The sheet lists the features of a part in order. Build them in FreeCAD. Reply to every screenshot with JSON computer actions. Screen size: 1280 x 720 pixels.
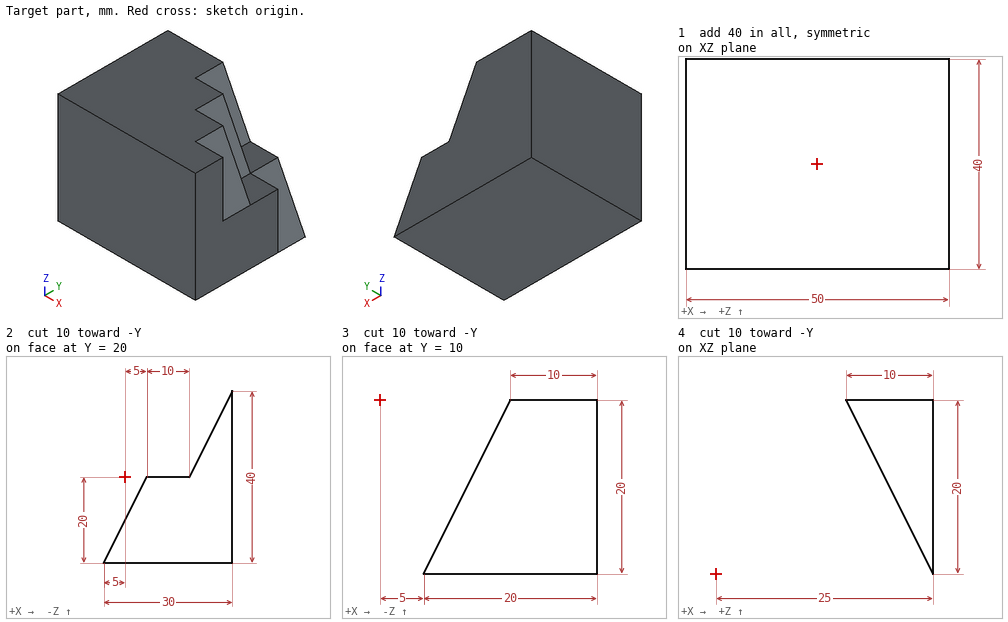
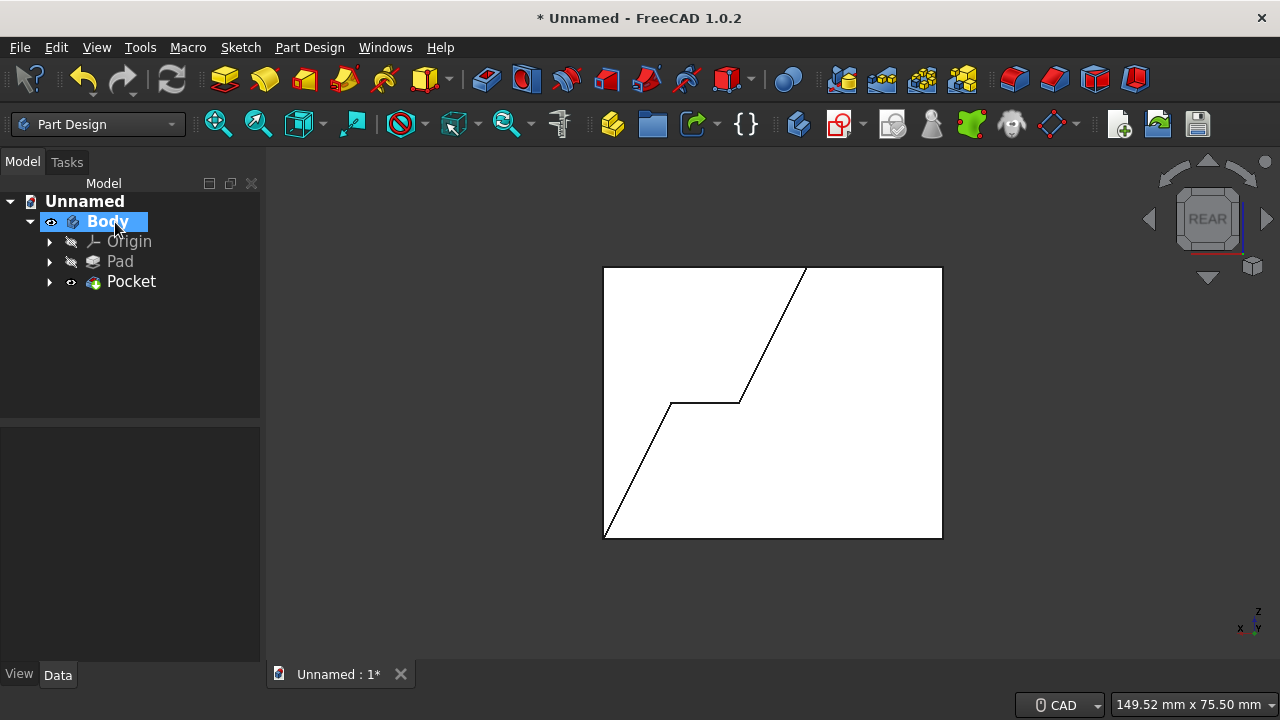
{"action": "left_click", "coordinate": [676, 324]}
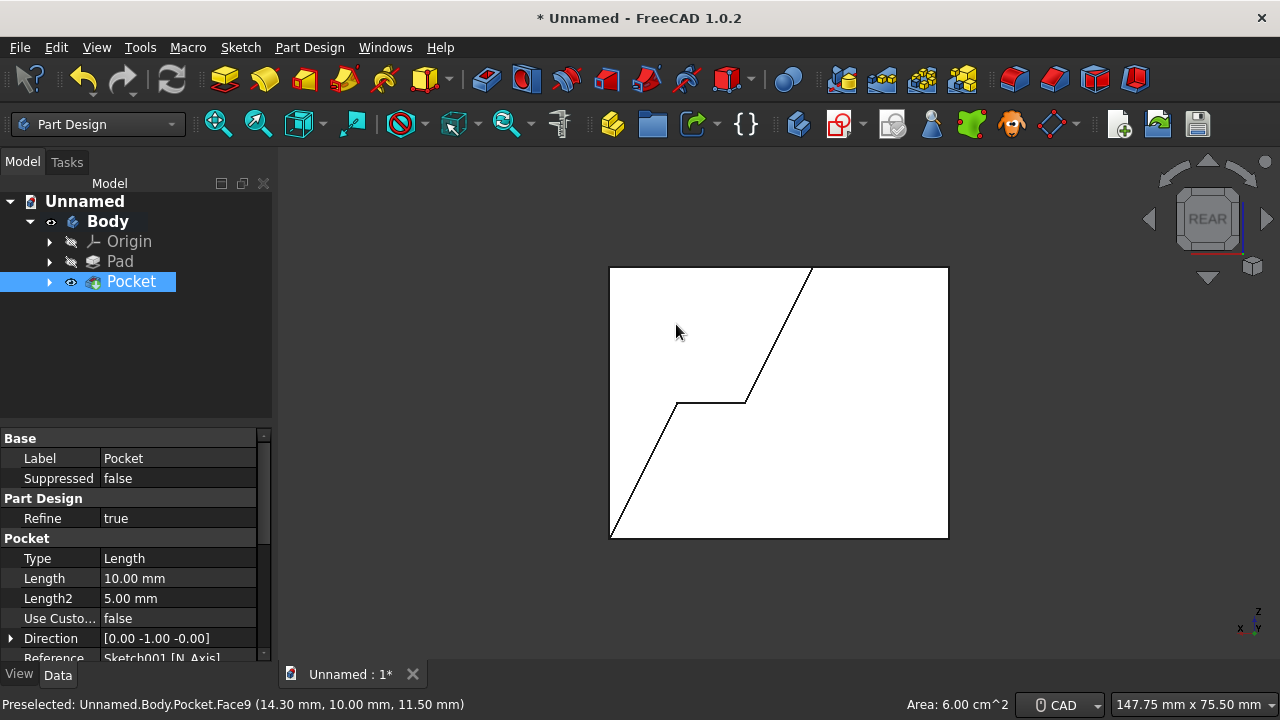
{"action": "left_click", "coordinate": [840, 124]}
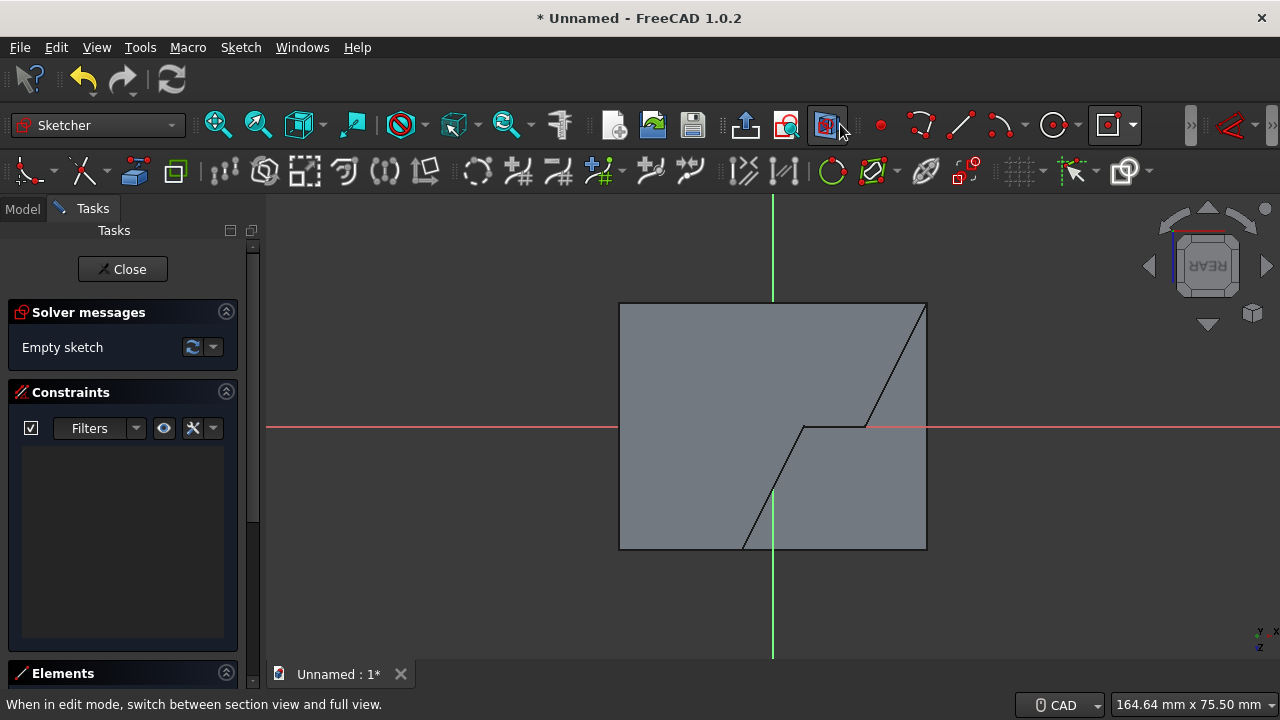
{"action": "scroll", "coordinate": [969, 538], "scroll_direction": "up", "scroll_amount": 4}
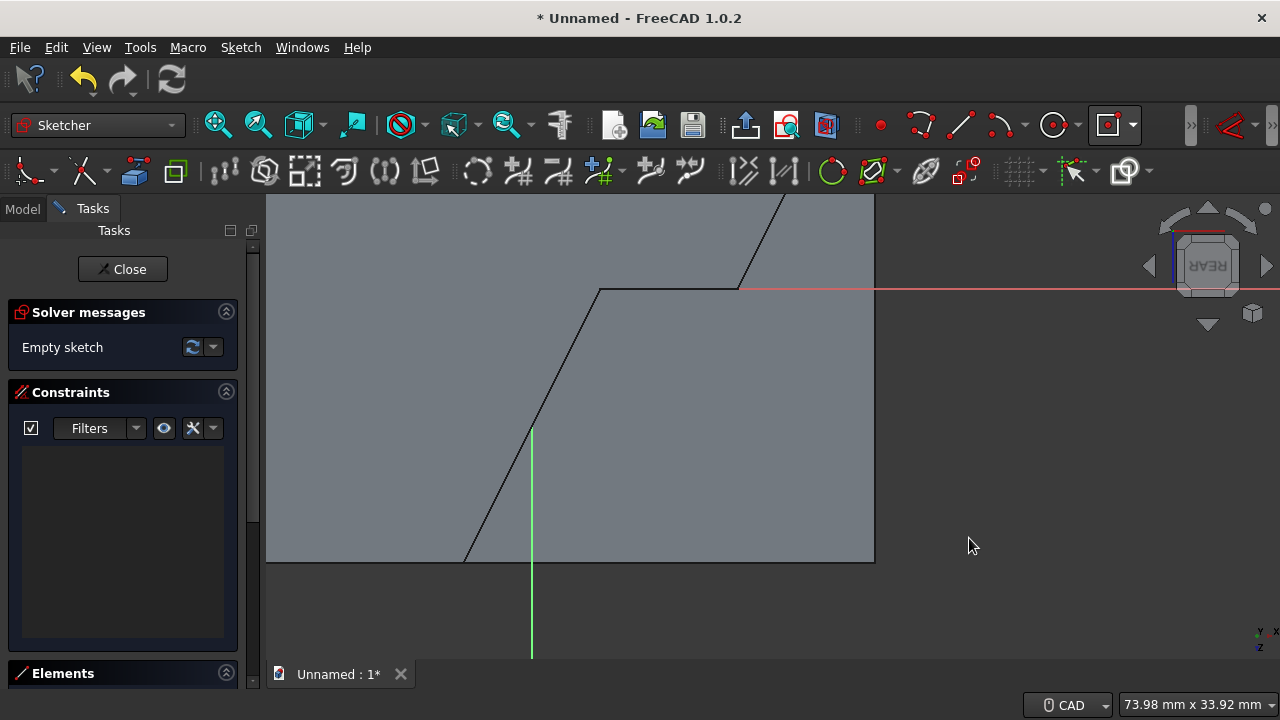
{"action": "left_click", "coordinate": [922, 126]}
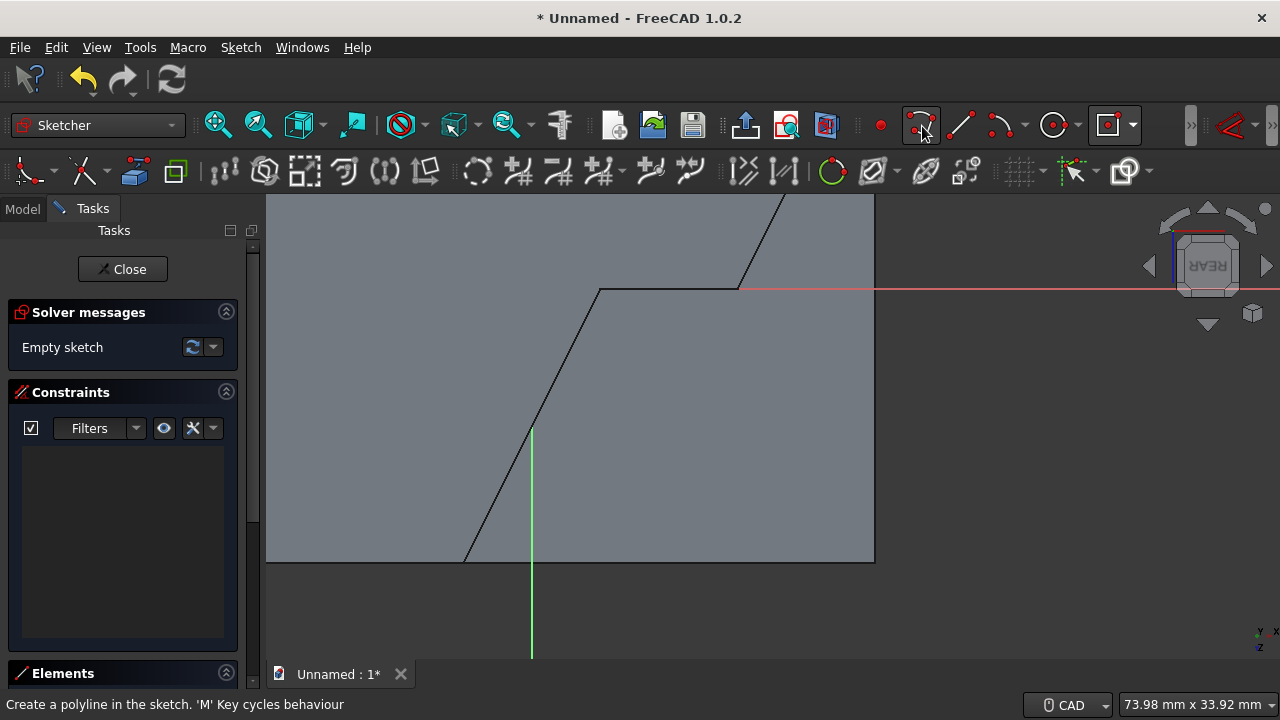
{"action": "left_click", "coordinate": [738, 289]}
{"action": "left_click", "coordinate": [600, 563]}
{"action": "left_click", "coordinate": [875, 563]}
{"action": "left_click", "coordinate": [875, 298]}
{"action": "left_click", "coordinate": [738, 289]}
{"action": "key", "text": "Escape"}
{"action": "key", "text": "Escape"}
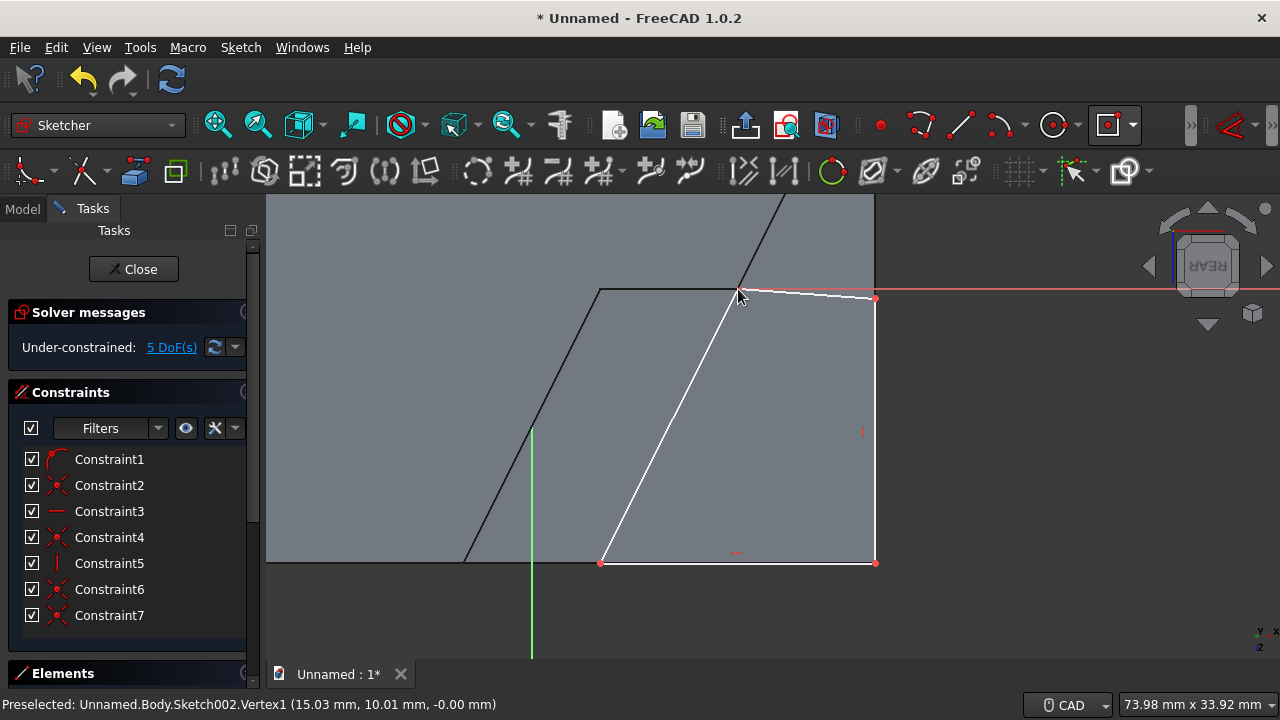
{"action": "left_click", "coordinate": [779, 292]}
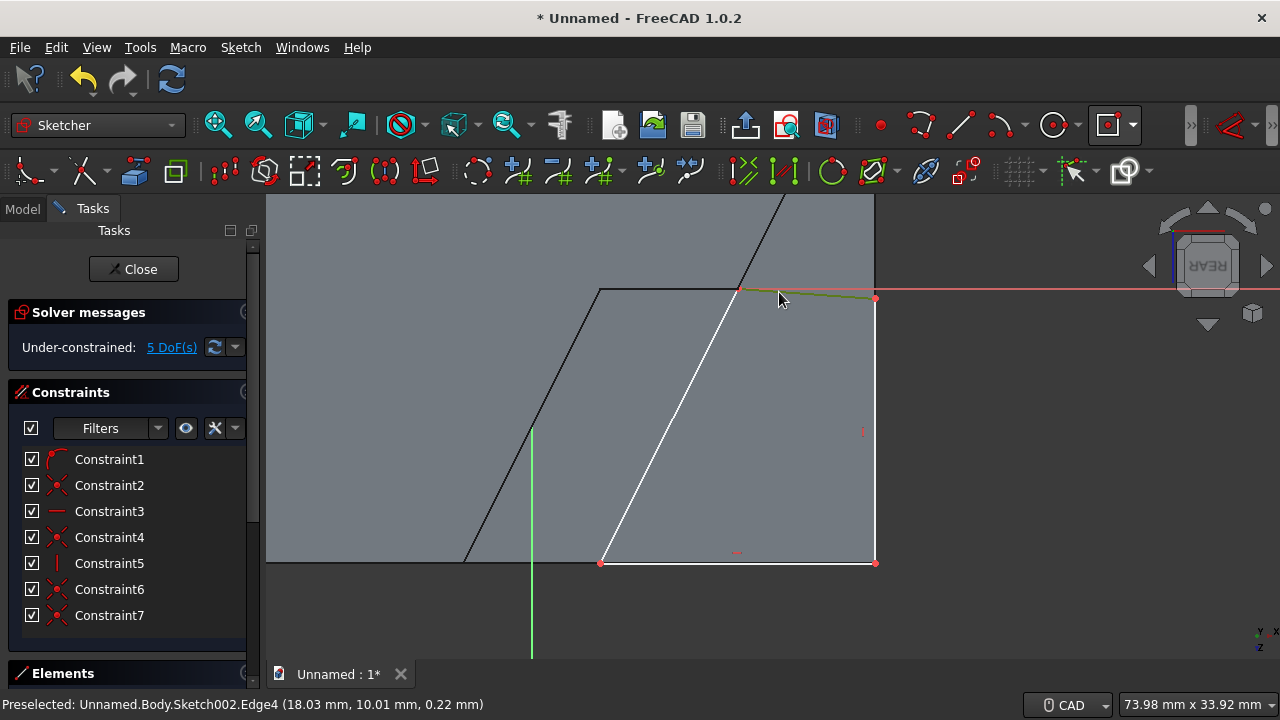
{"action": "key", "text": "h"}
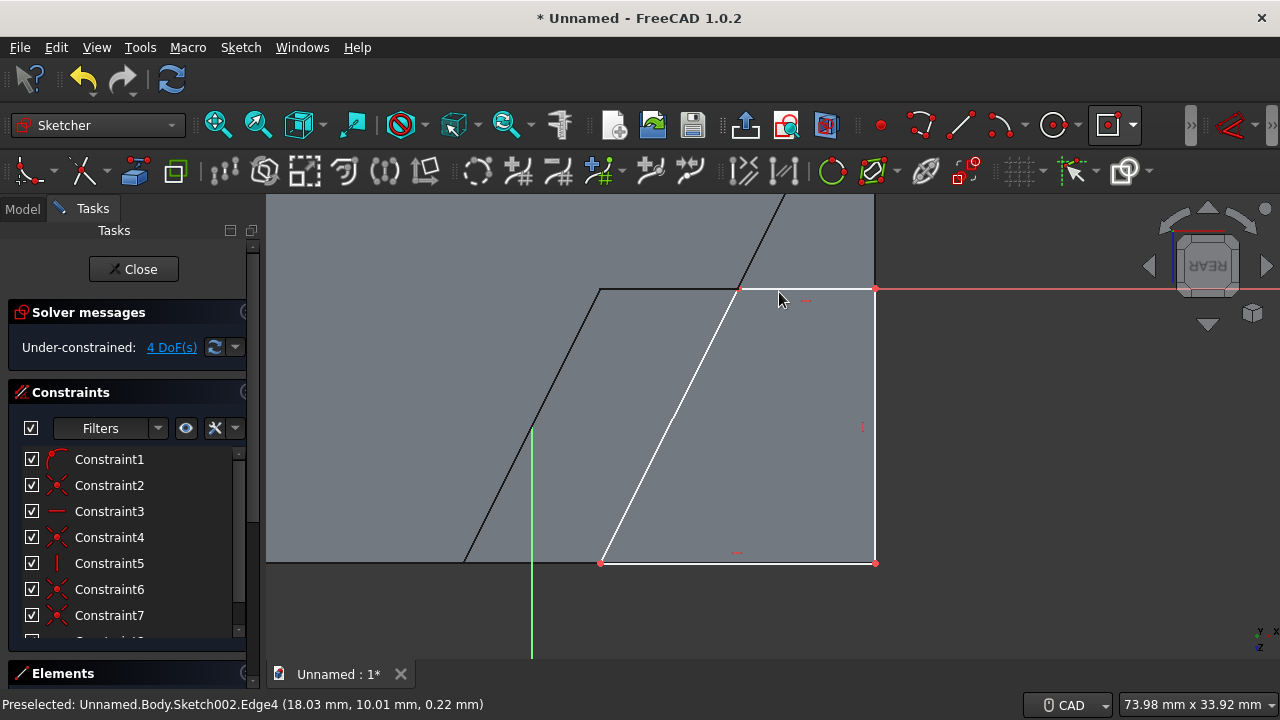
{"action": "left_click", "coordinate": [1230, 126]}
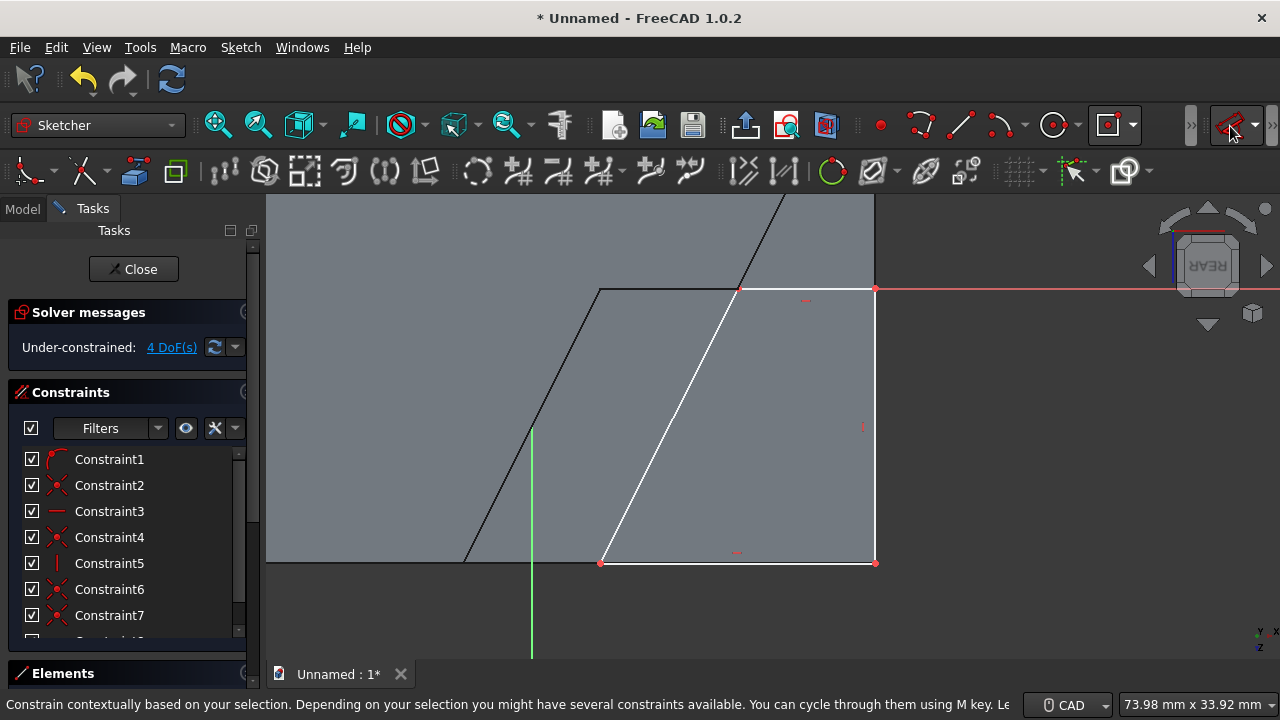
{"action": "left_click", "coordinate": [682, 564]}
{"action": "left_click", "coordinate": [738, 598]}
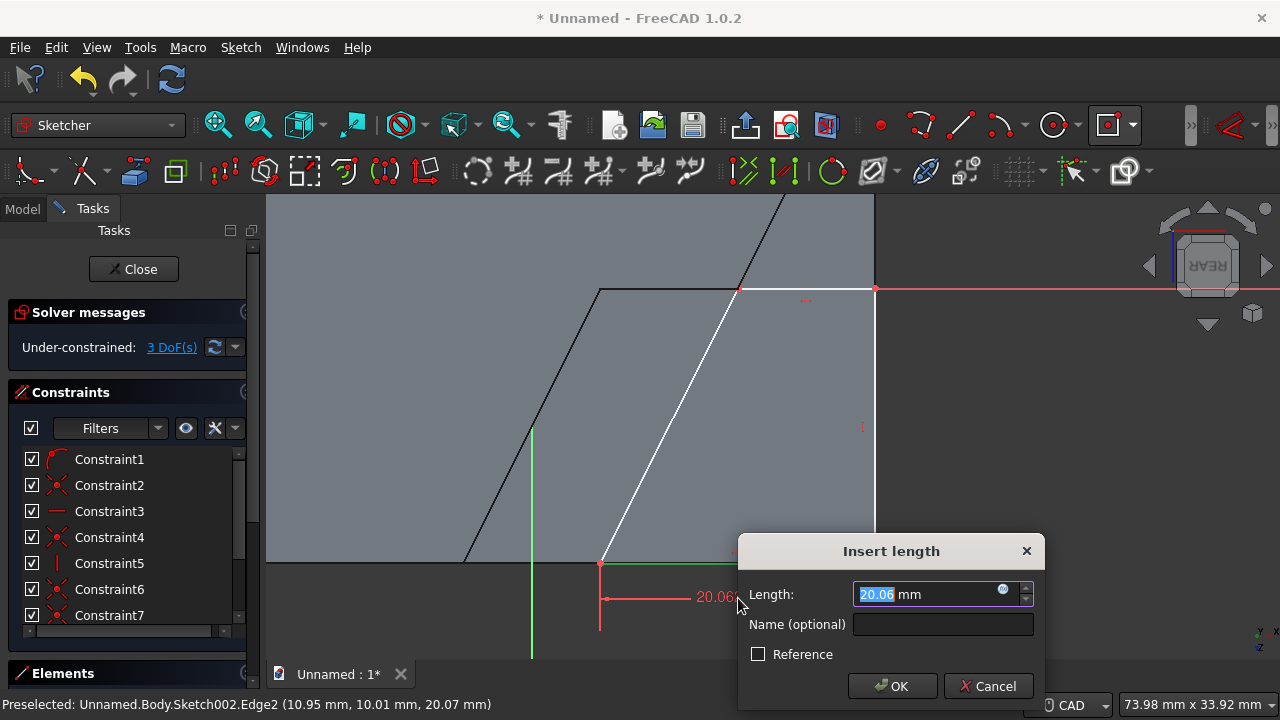
{"action": "type", "text": "20"}
{"action": "key", "text": "Return"}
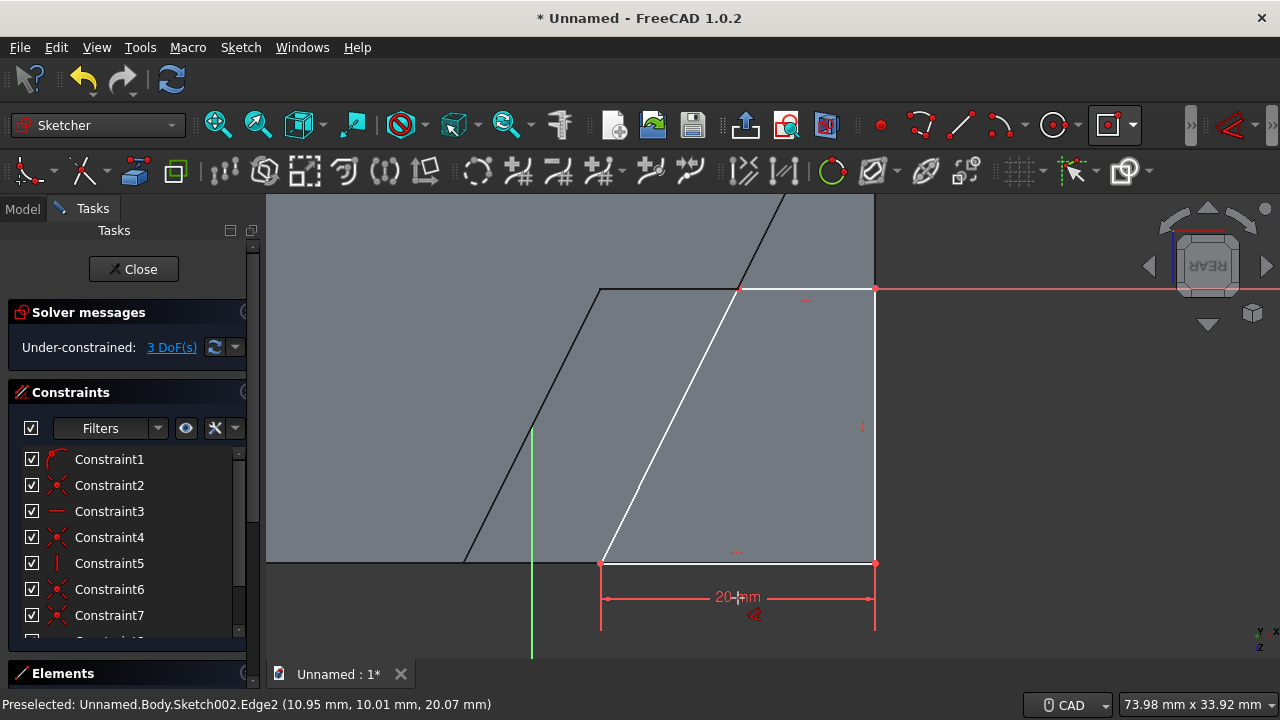
{"action": "left_click", "coordinate": [875, 481]}
{"action": "left_click", "coordinate": [909, 426]}